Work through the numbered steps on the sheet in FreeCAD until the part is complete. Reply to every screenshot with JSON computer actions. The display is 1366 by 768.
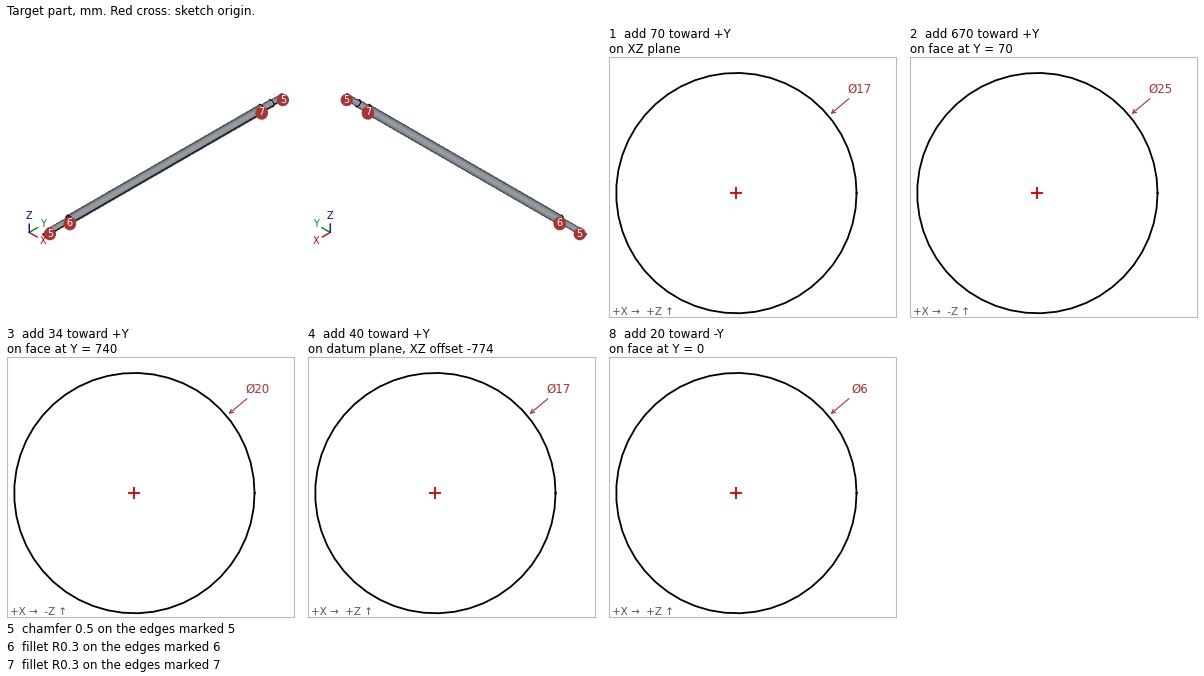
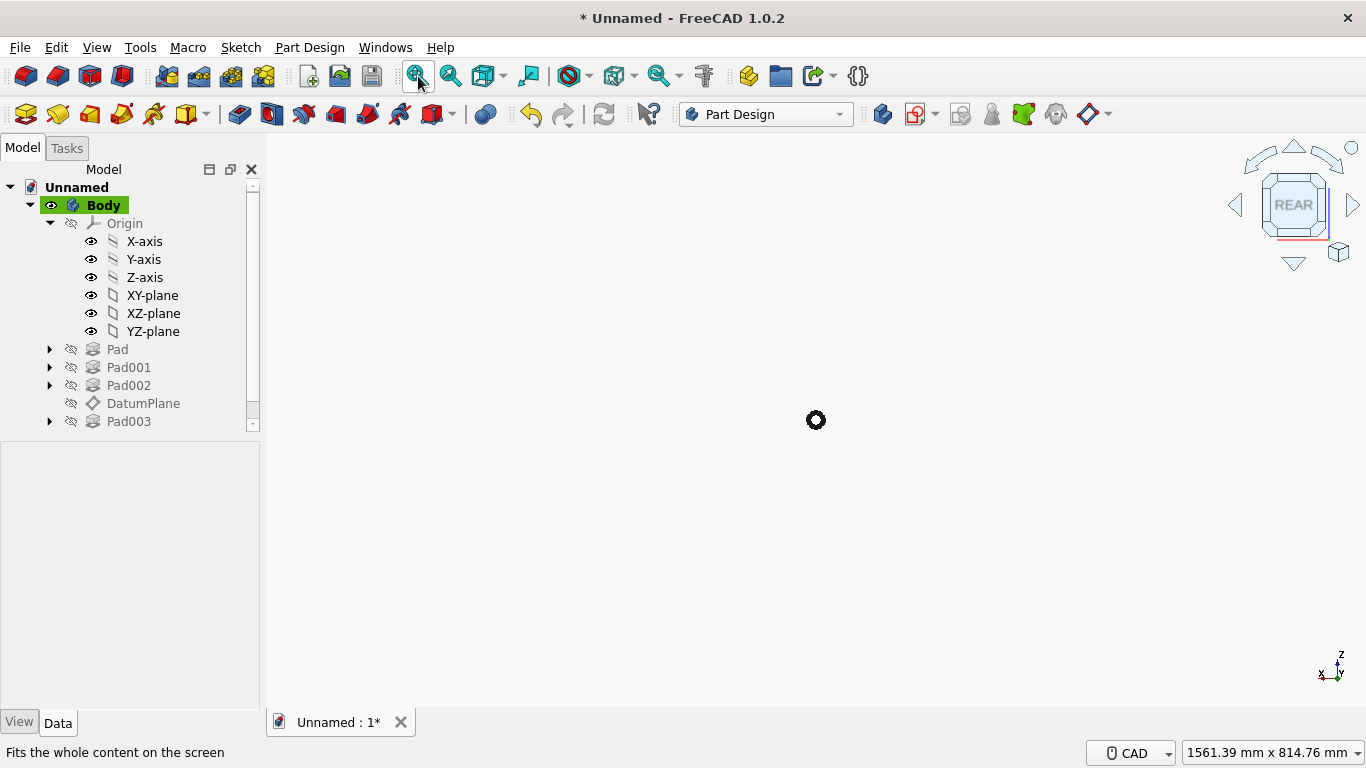
{"action": "left_click", "coordinate": [418, 76]}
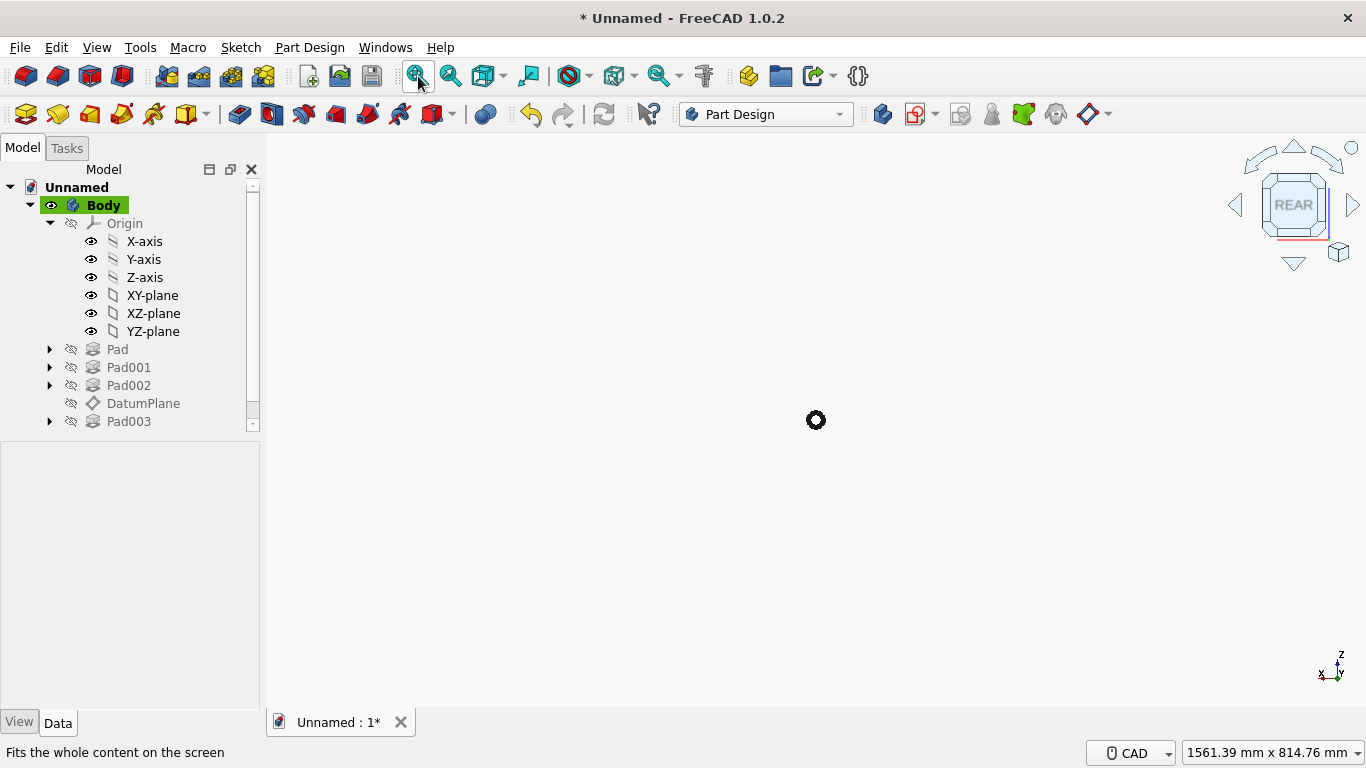
{"action": "key", "text": "6"}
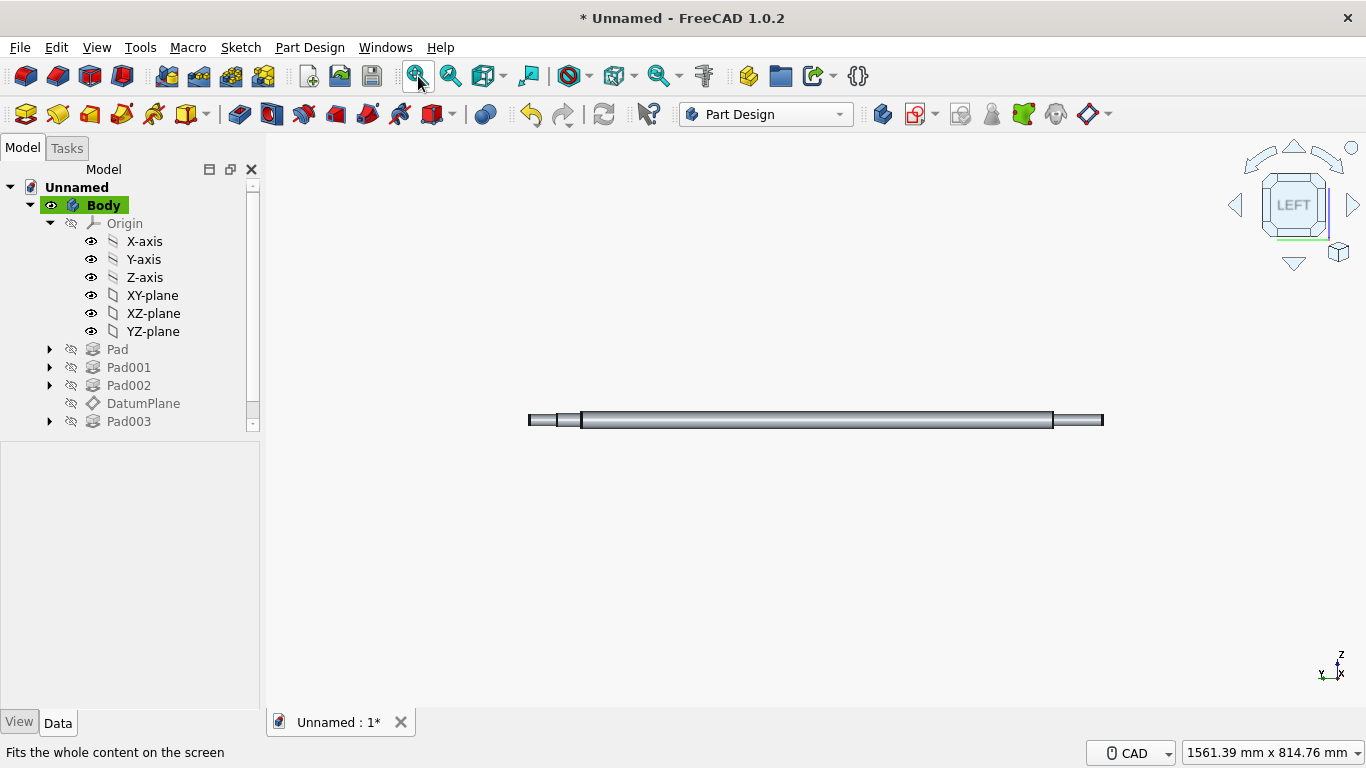
{"action": "key", "text": "v 3"}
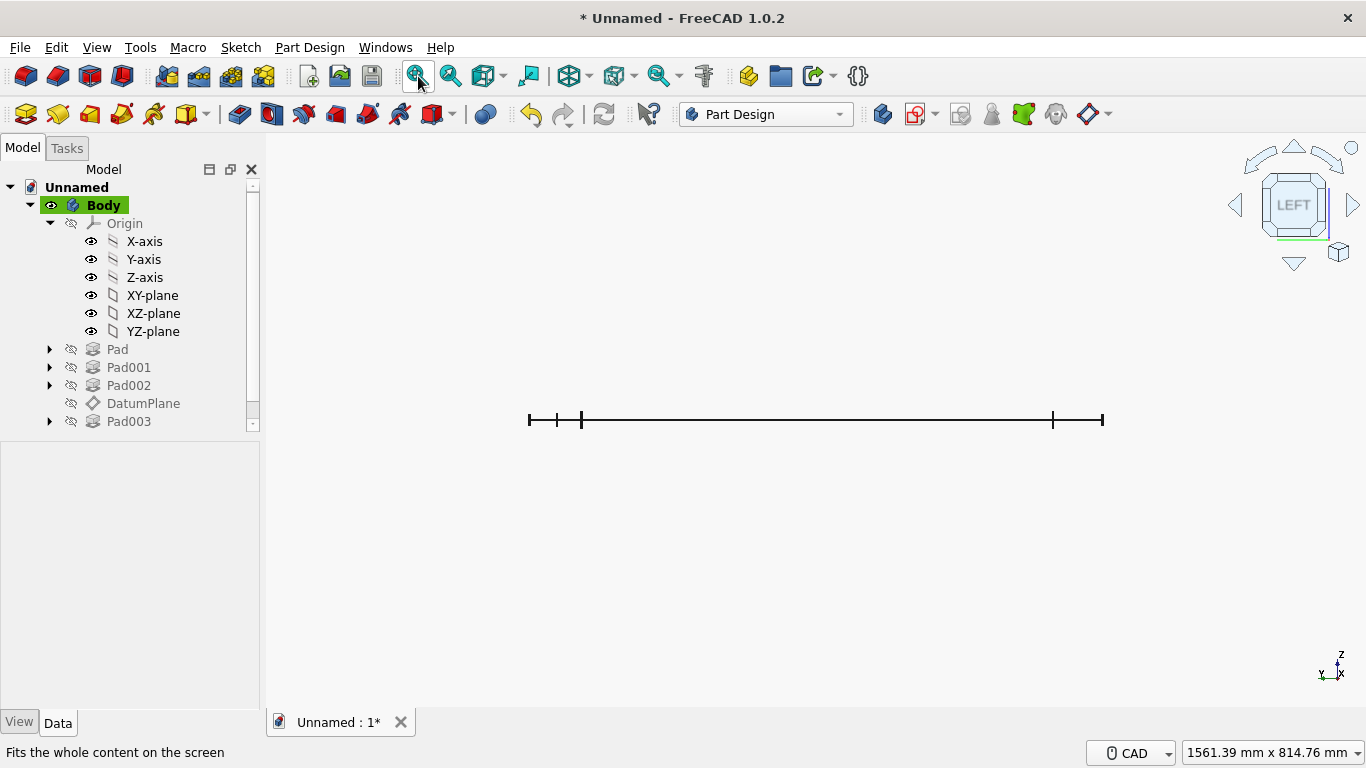
{"action": "key", "text": "0"}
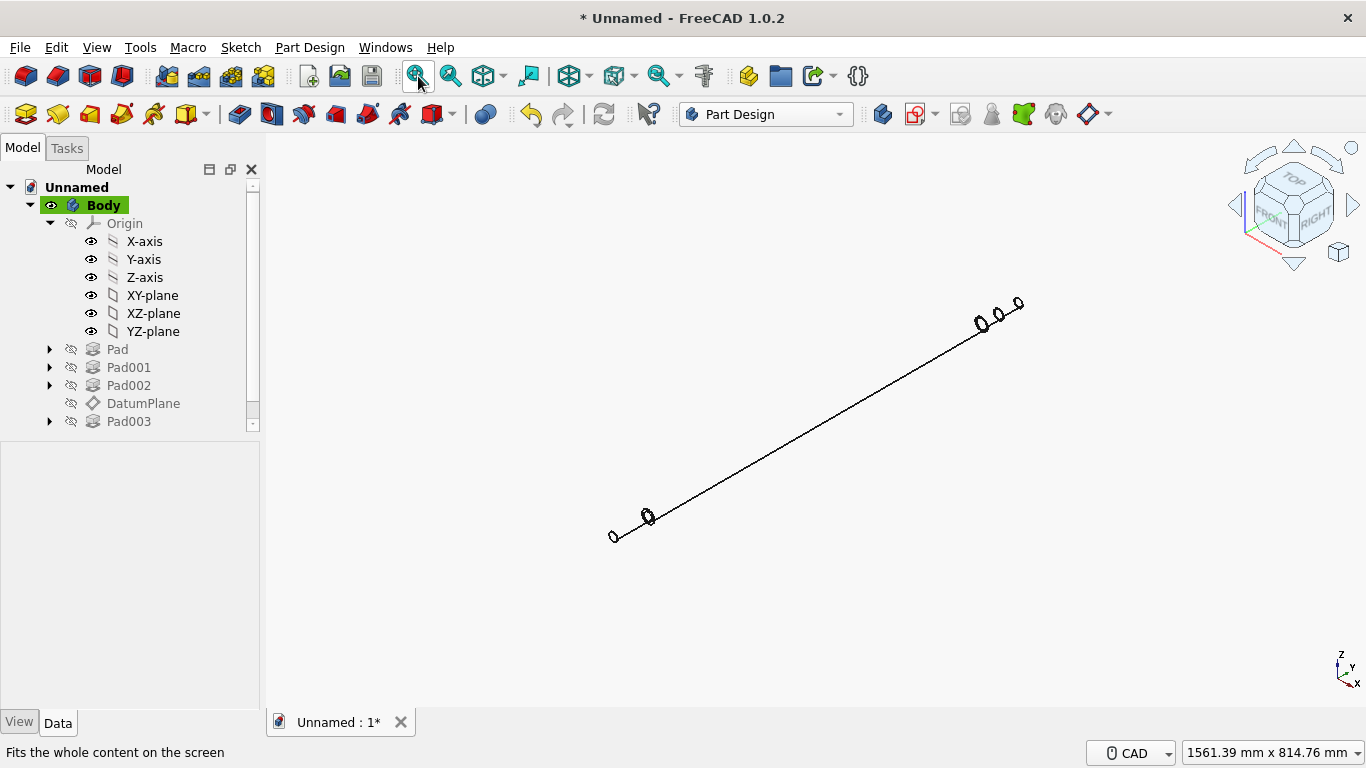
{"action": "left_click", "coordinate": [418, 76]}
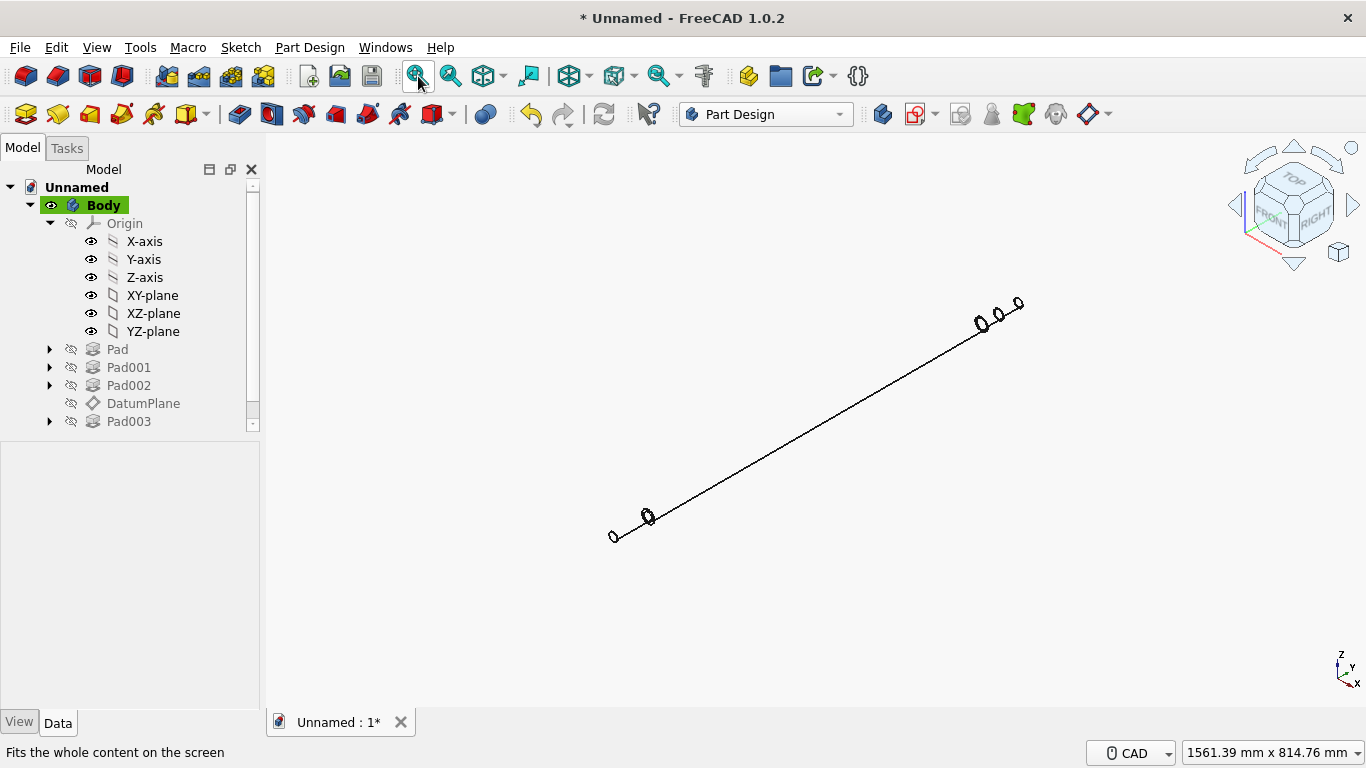
{"action": "scroll", "coordinate": [644, 513], "scroll_direction": "up", "scroll_amount": 6}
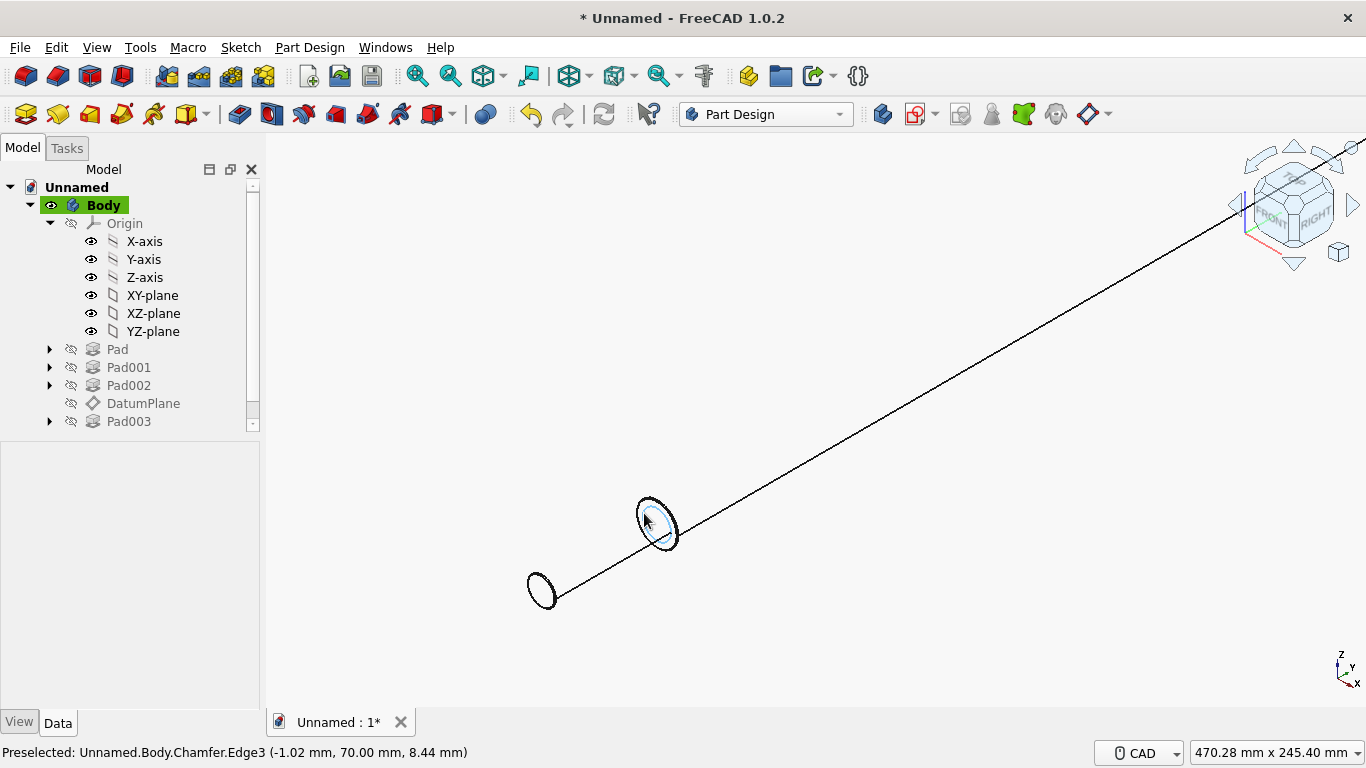
{"action": "left_click", "coordinate": [643, 515]}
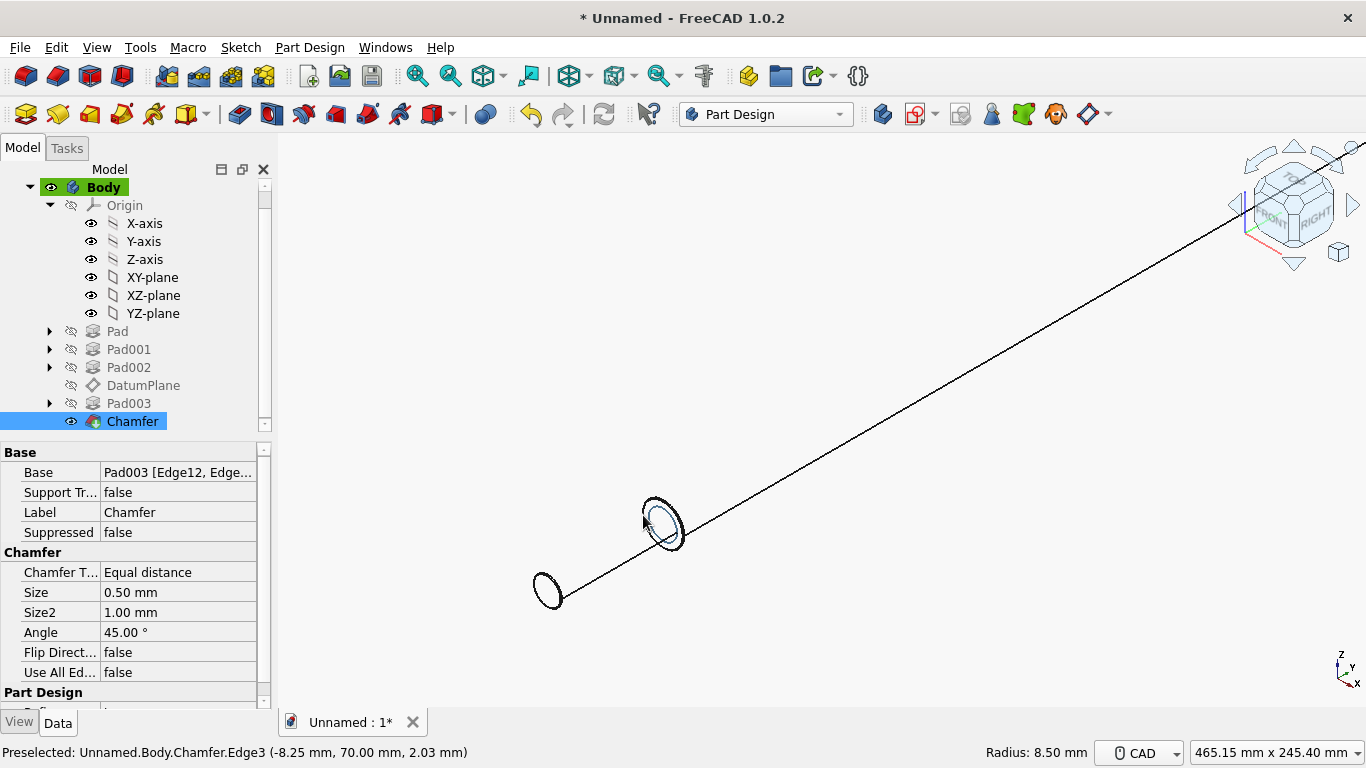
{"action": "key", "text": "v 1"}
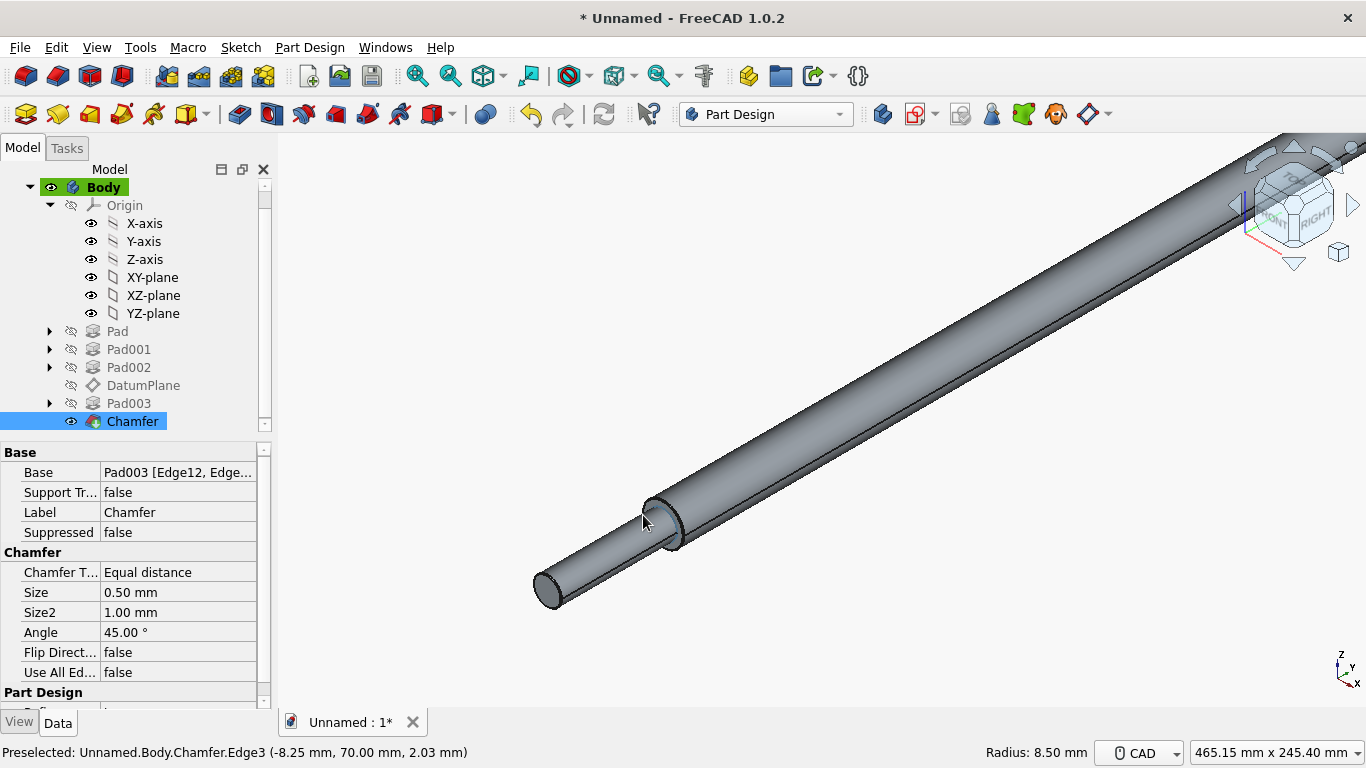
{"action": "left_click", "coordinate": [26, 76]}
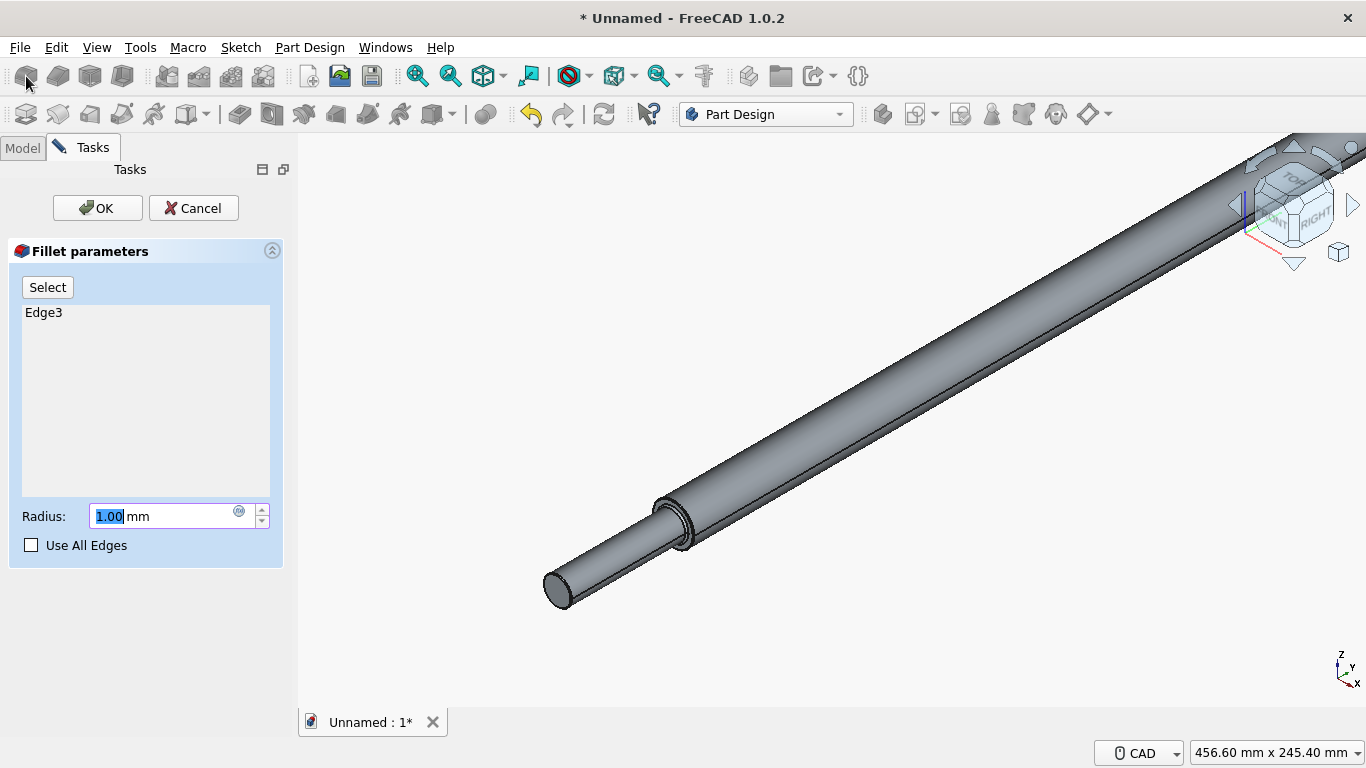
{"action": "type", "text": "0.3"}
{"action": "key", "text": "Tab"}